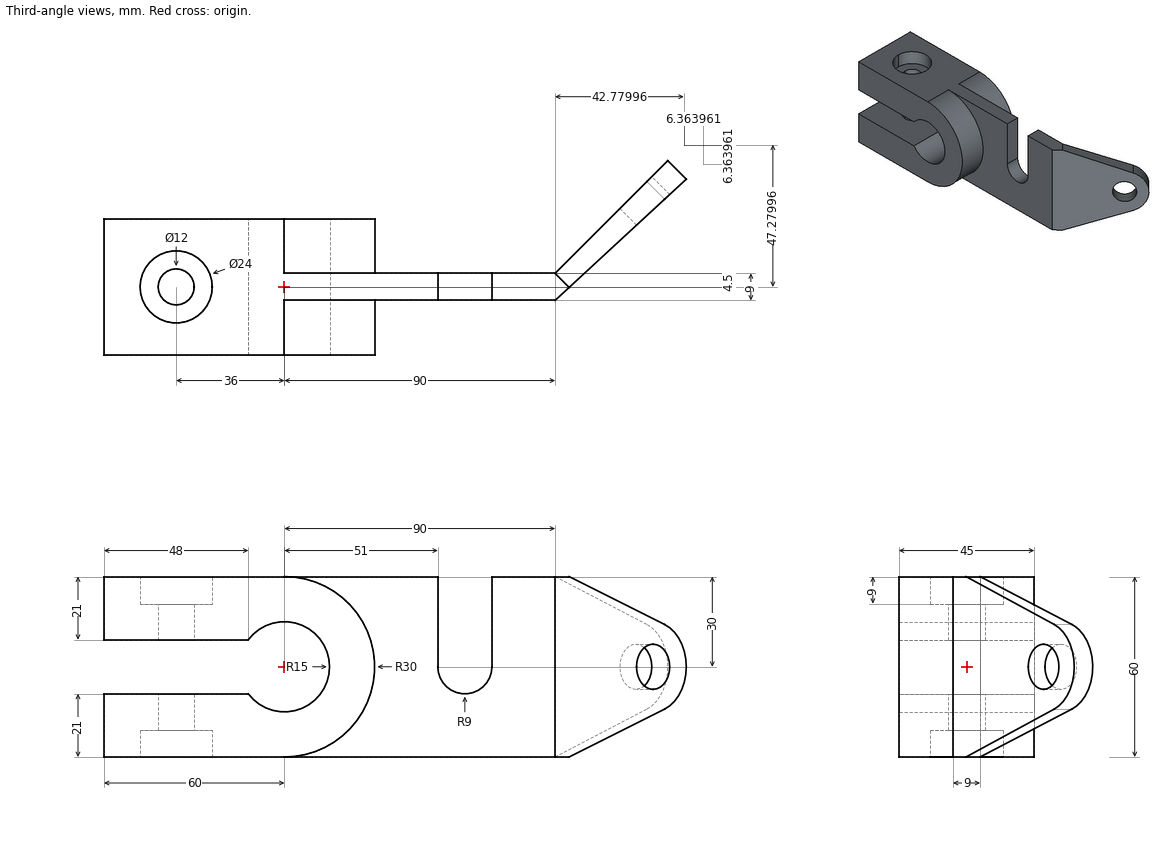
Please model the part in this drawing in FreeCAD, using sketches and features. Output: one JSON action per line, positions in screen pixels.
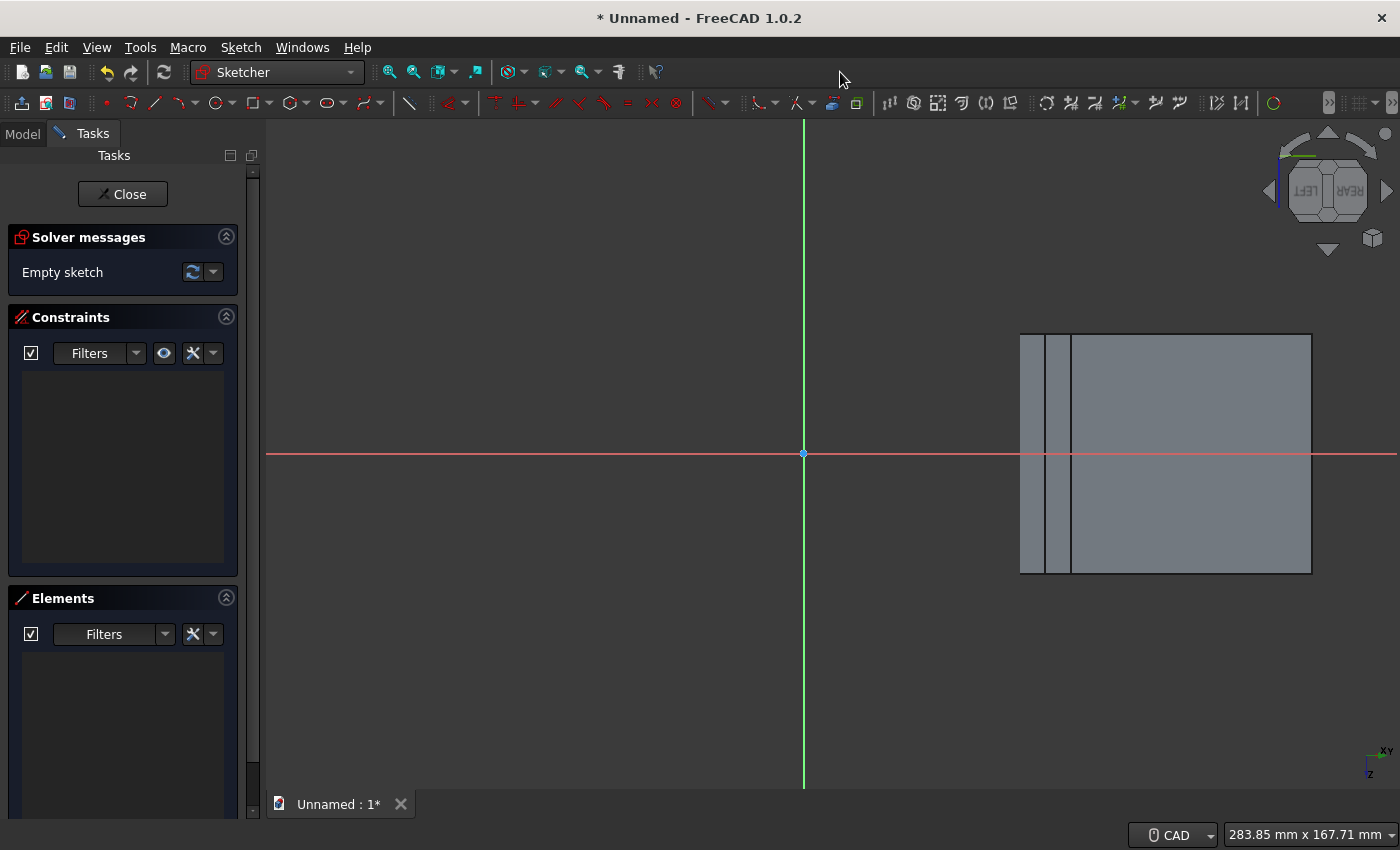
{"action": "scroll", "coordinate": [294, 454], "scroll_direction": "down", "scroll_amount": 1}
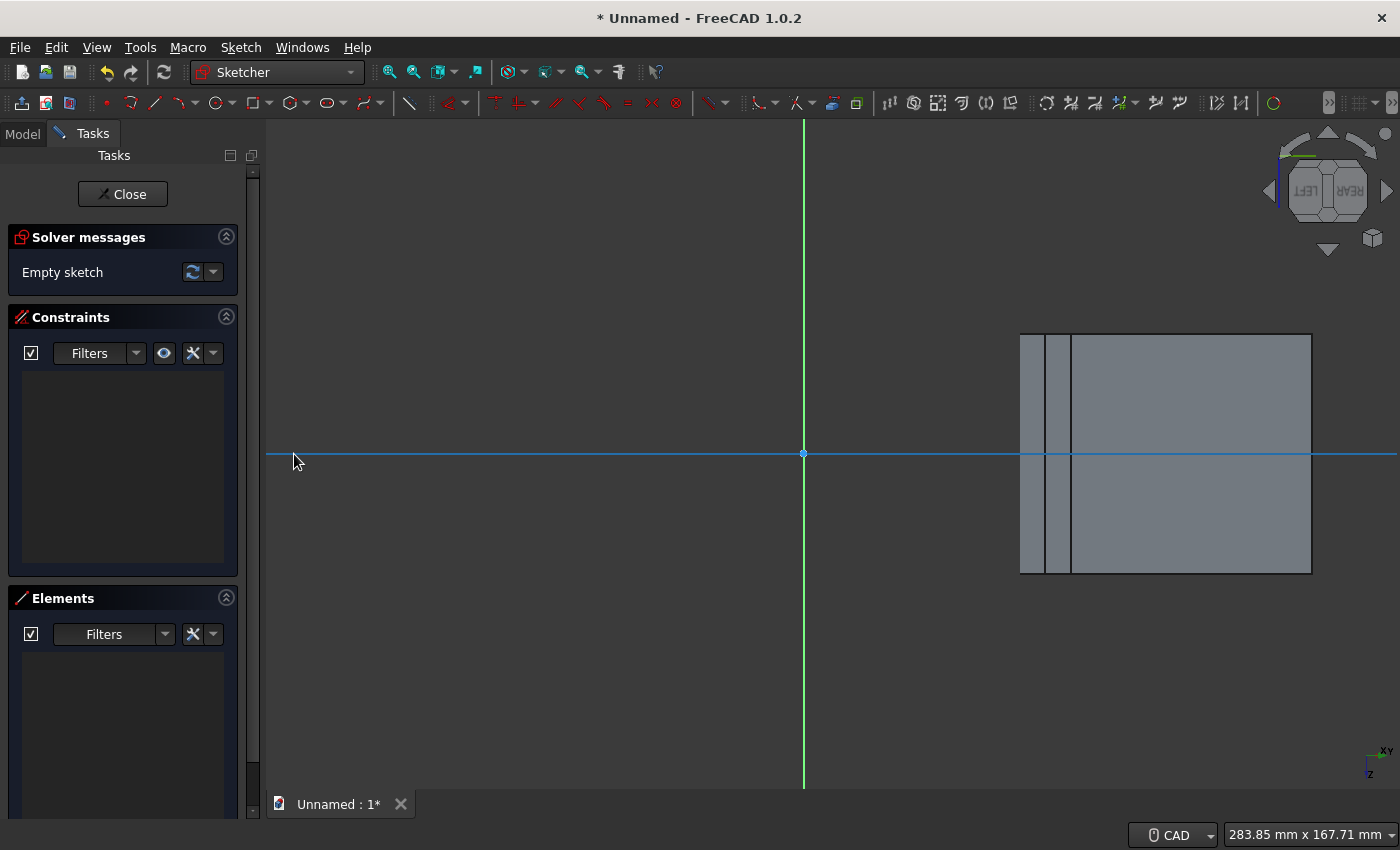
{"action": "scroll", "coordinate": [1235, 454], "scroll_direction": "up", "scroll_amount": 2}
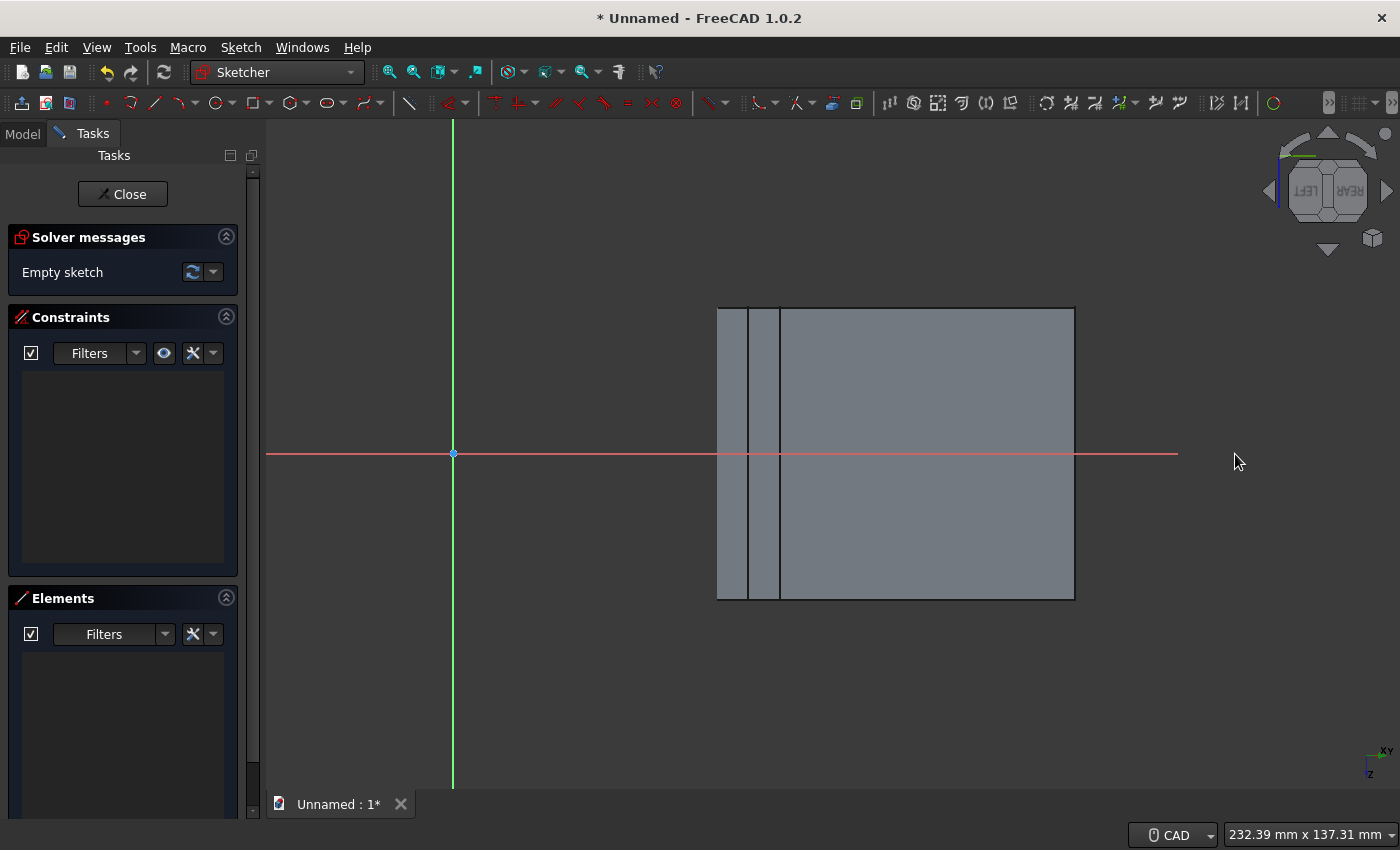
{"action": "left_click", "coordinate": [132, 104]}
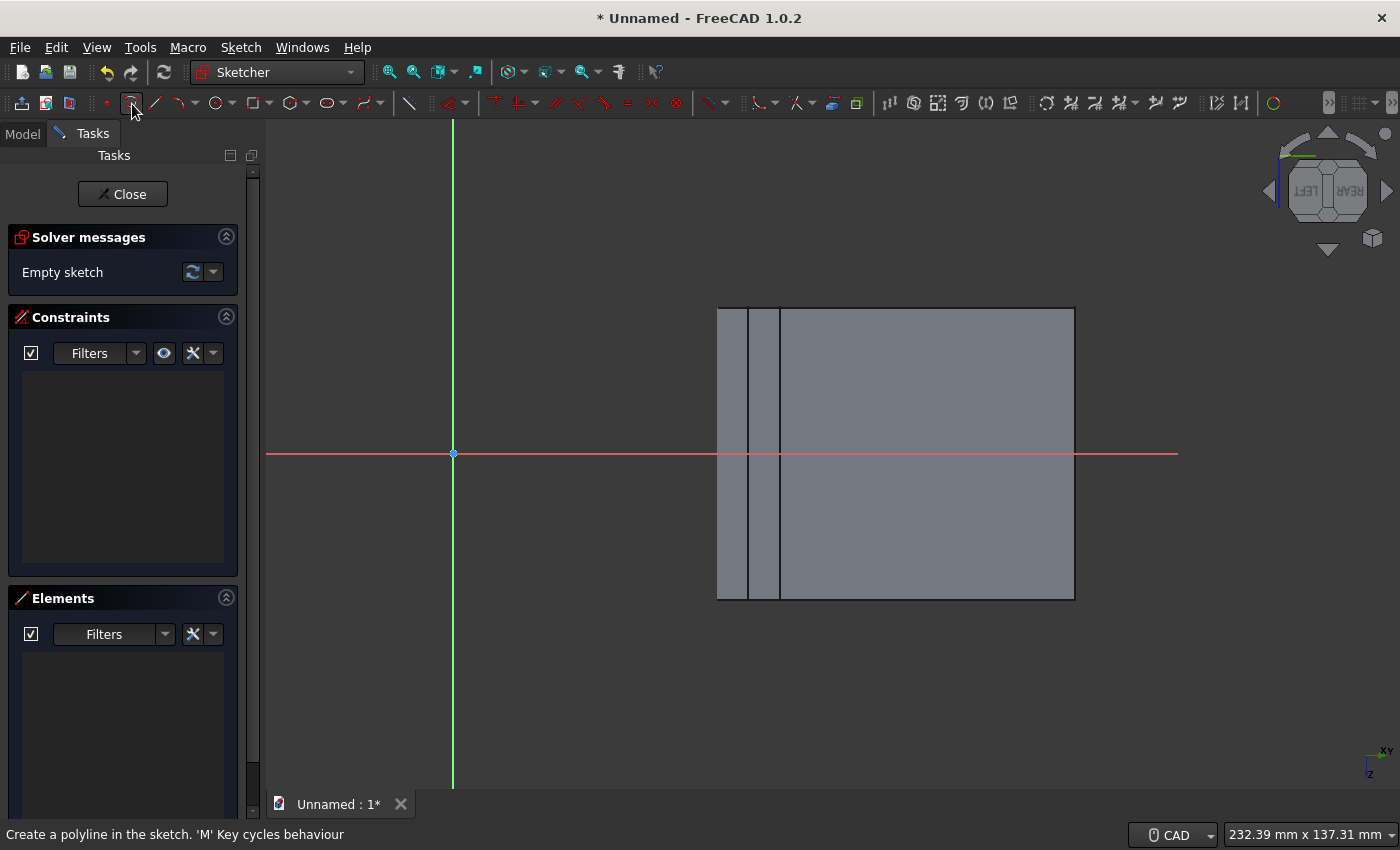
{"action": "left_click", "coordinate": [990, 523]}
{"action": "left_click", "coordinate": [780, 600]}
{"action": "left_click", "coordinate": [1075, 600]}
{"action": "left_click", "coordinate": [1075, 308]}
{"action": "left_click", "coordinate": [780, 308]}
{"action": "left_click", "coordinate": [990, 385]}
{"action": "right_click", "coordinate": [990, 385]}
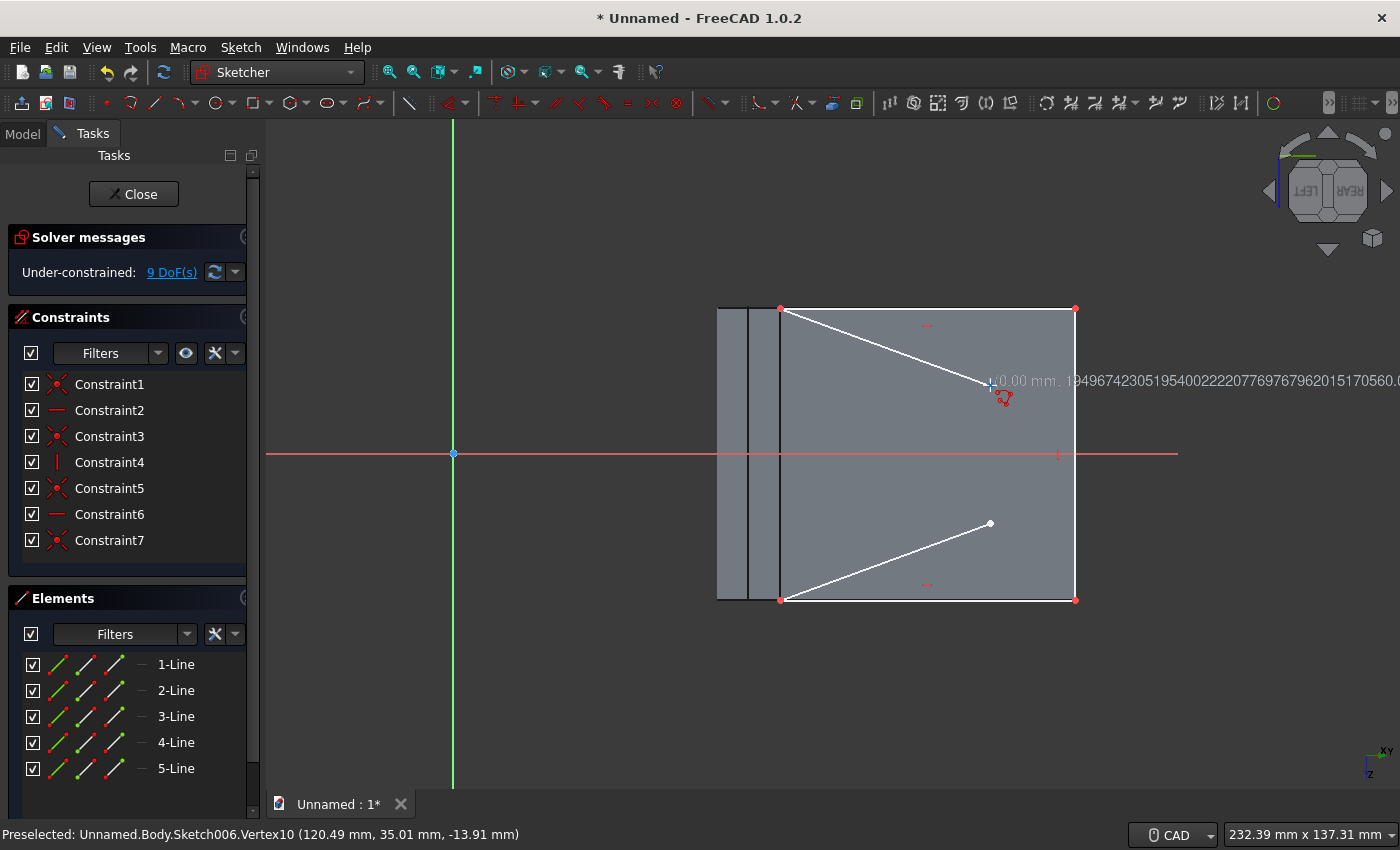
{"action": "key", "text": "g 3 a"}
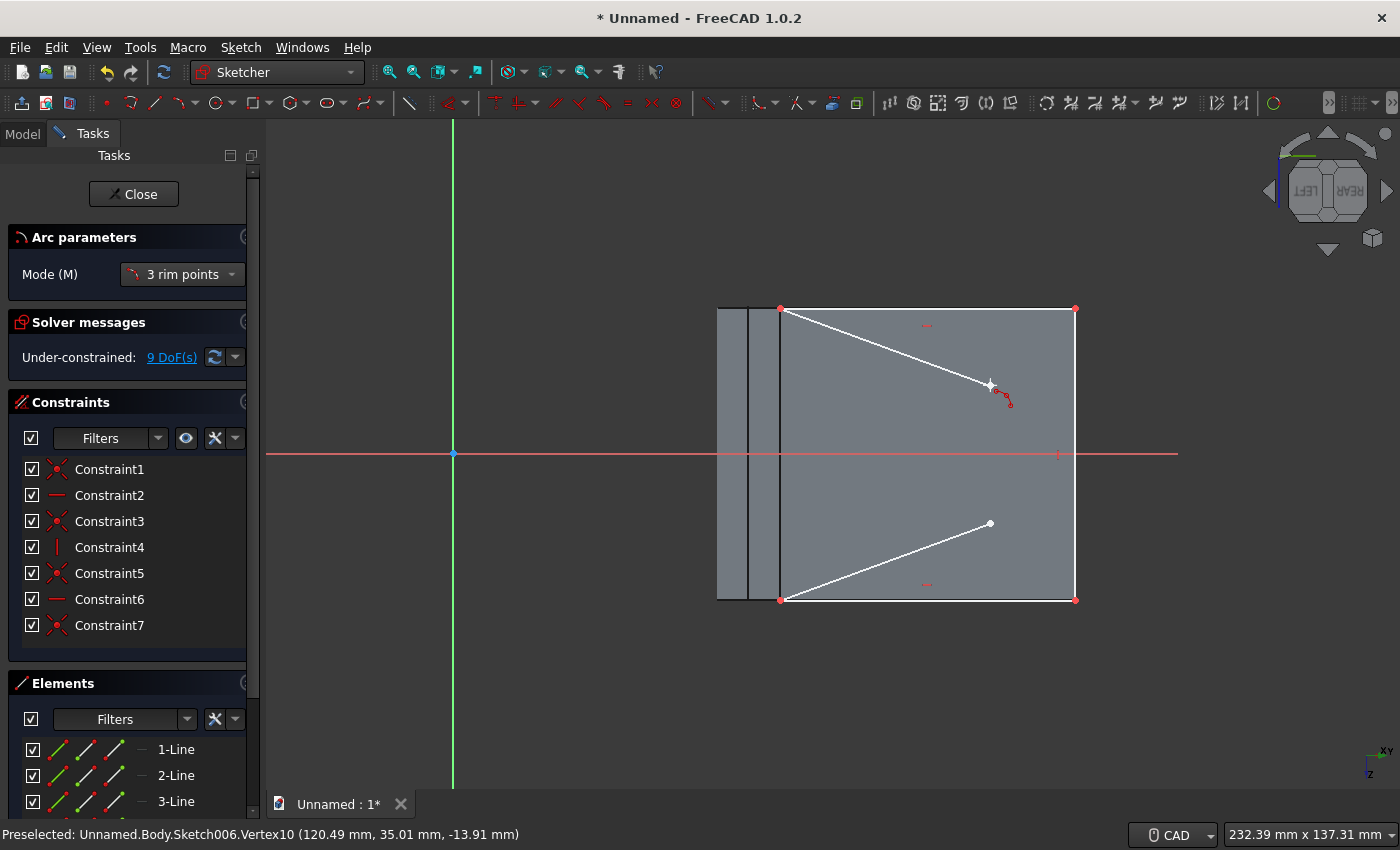
{"action": "left_click", "coordinate": [990, 386]}
{"action": "left_click", "coordinate": [990, 524]}
{"action": "left_click", "coordinate": [1036, 472]}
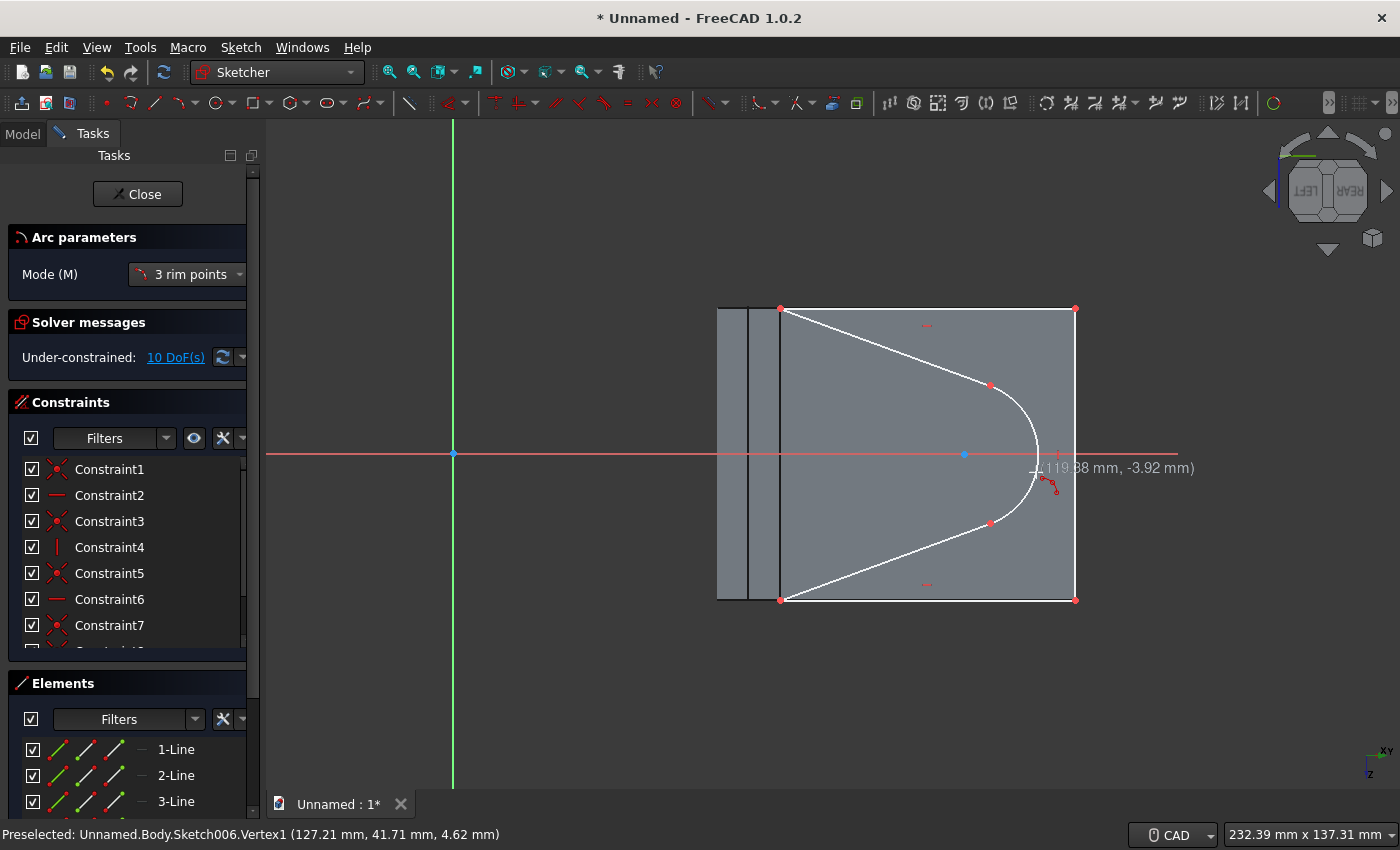
{"action": "key", "text": "g c"}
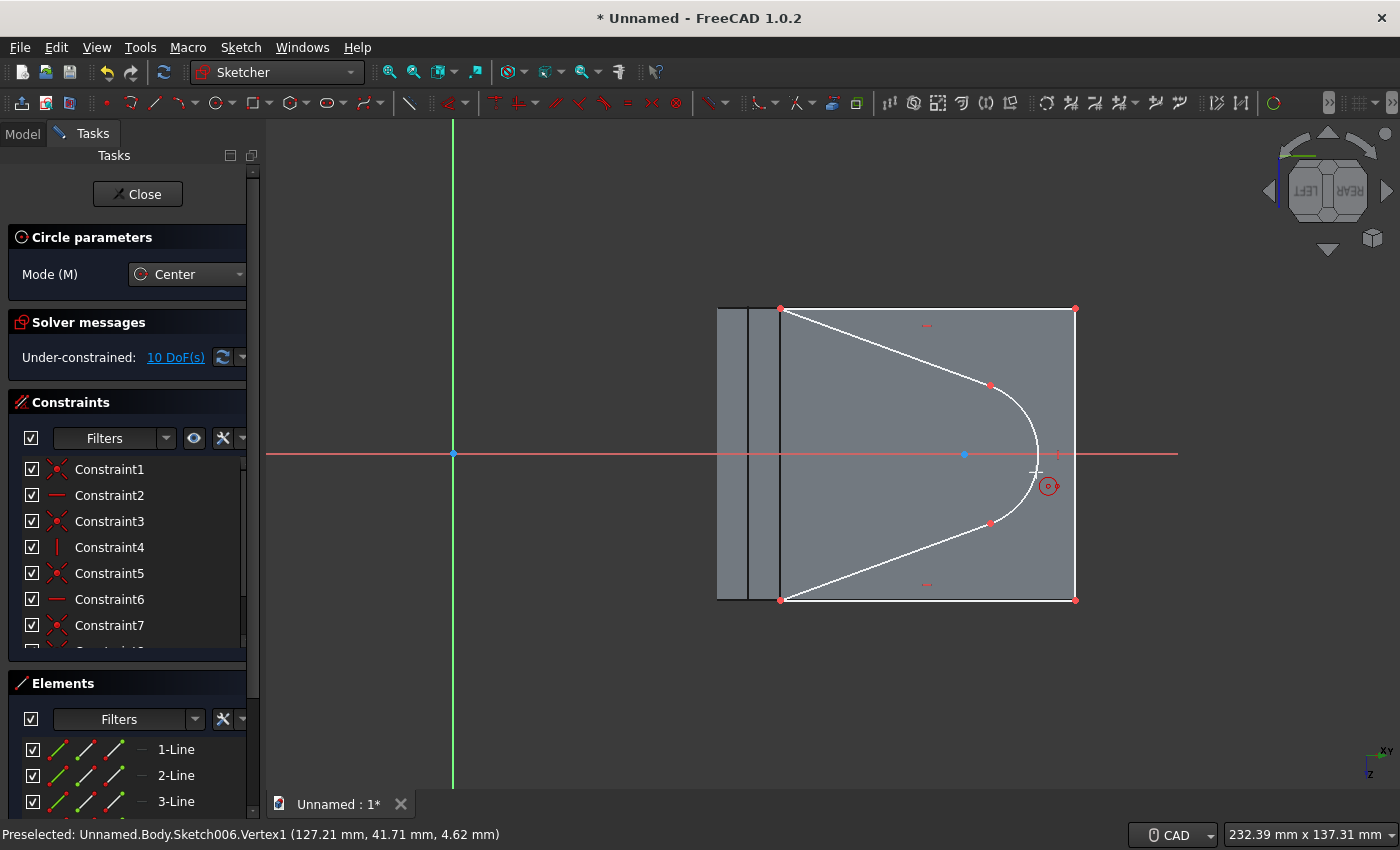
{"action": "left_click", "coordinate": [965, 454]}
{"action": "left_click", "coordinate": [991, 428]}
{"action": "key", "text": "Escape"}